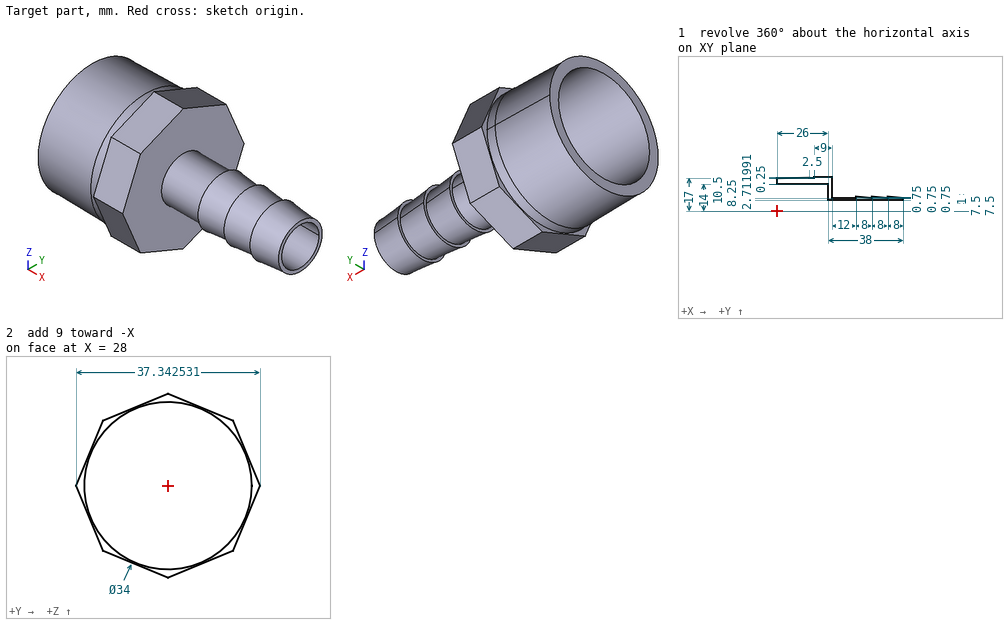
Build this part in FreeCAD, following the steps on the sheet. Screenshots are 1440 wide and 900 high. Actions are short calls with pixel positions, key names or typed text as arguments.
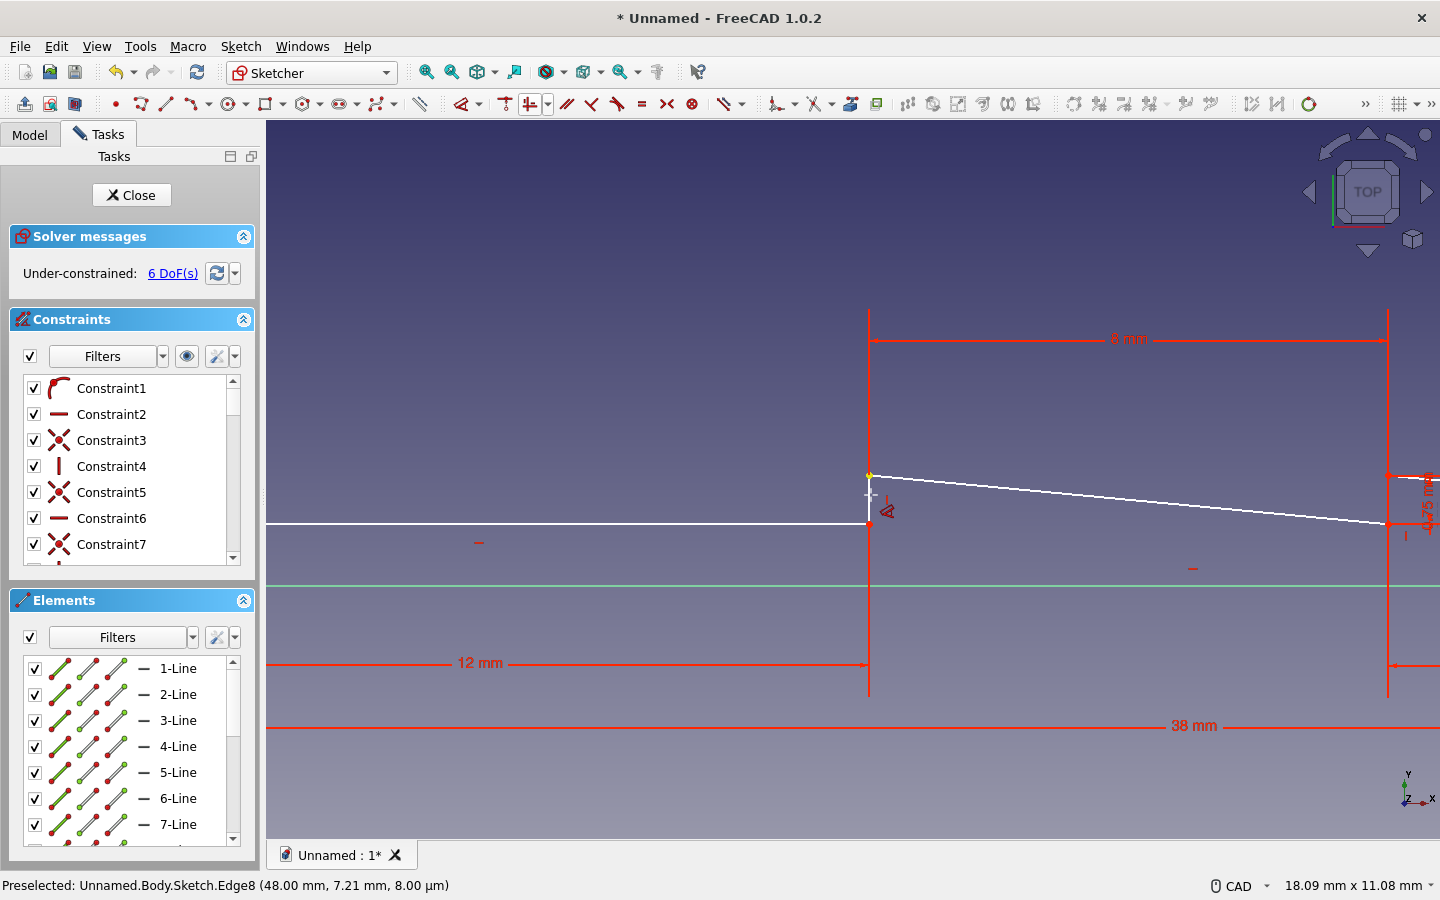
click(869, 490)
click(903, 500)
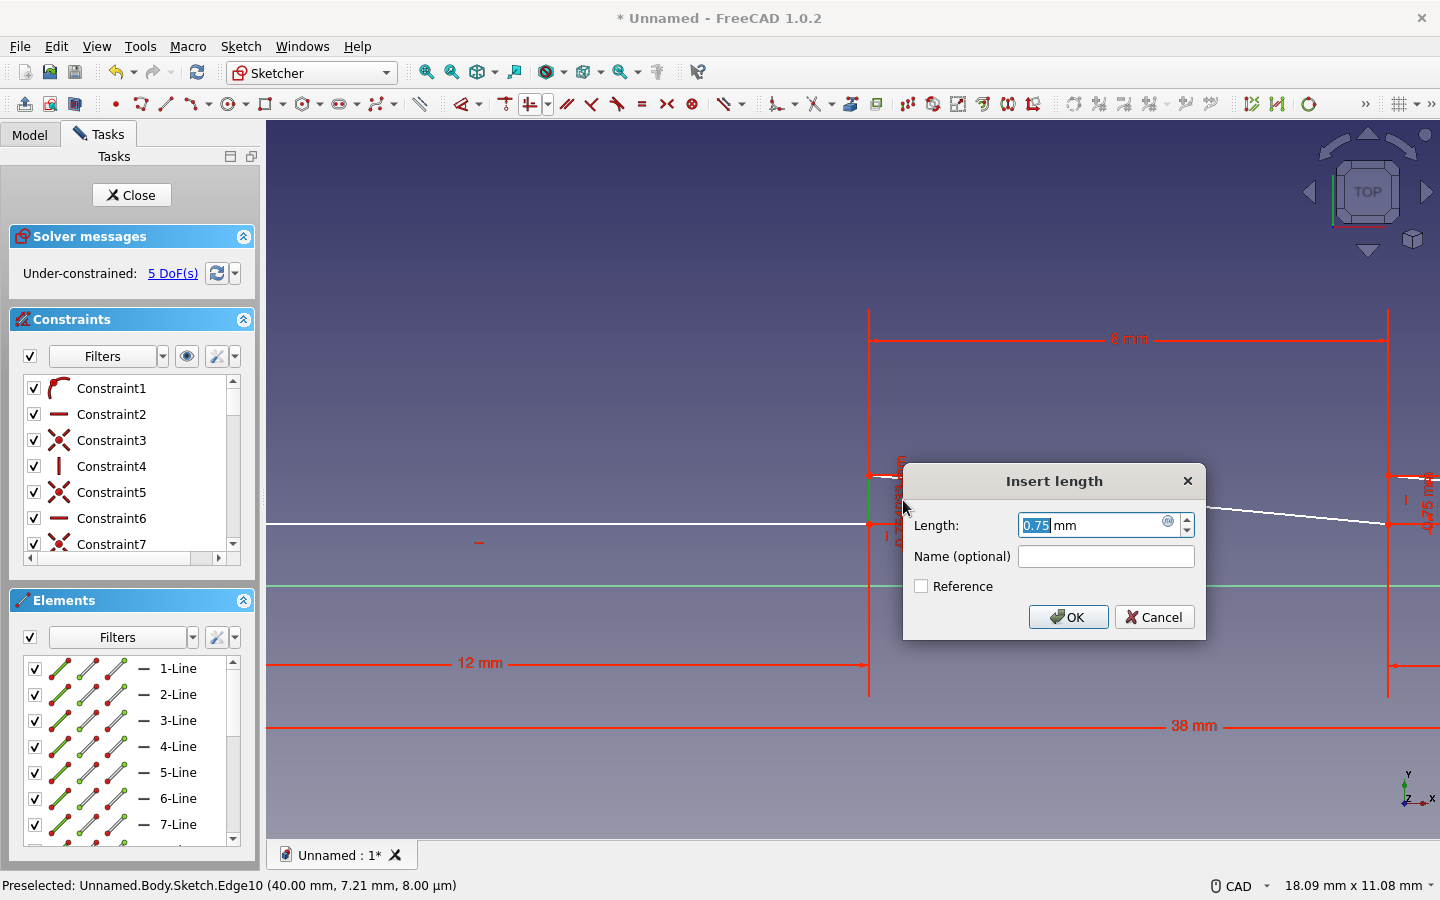
text(0.75)
key(Return)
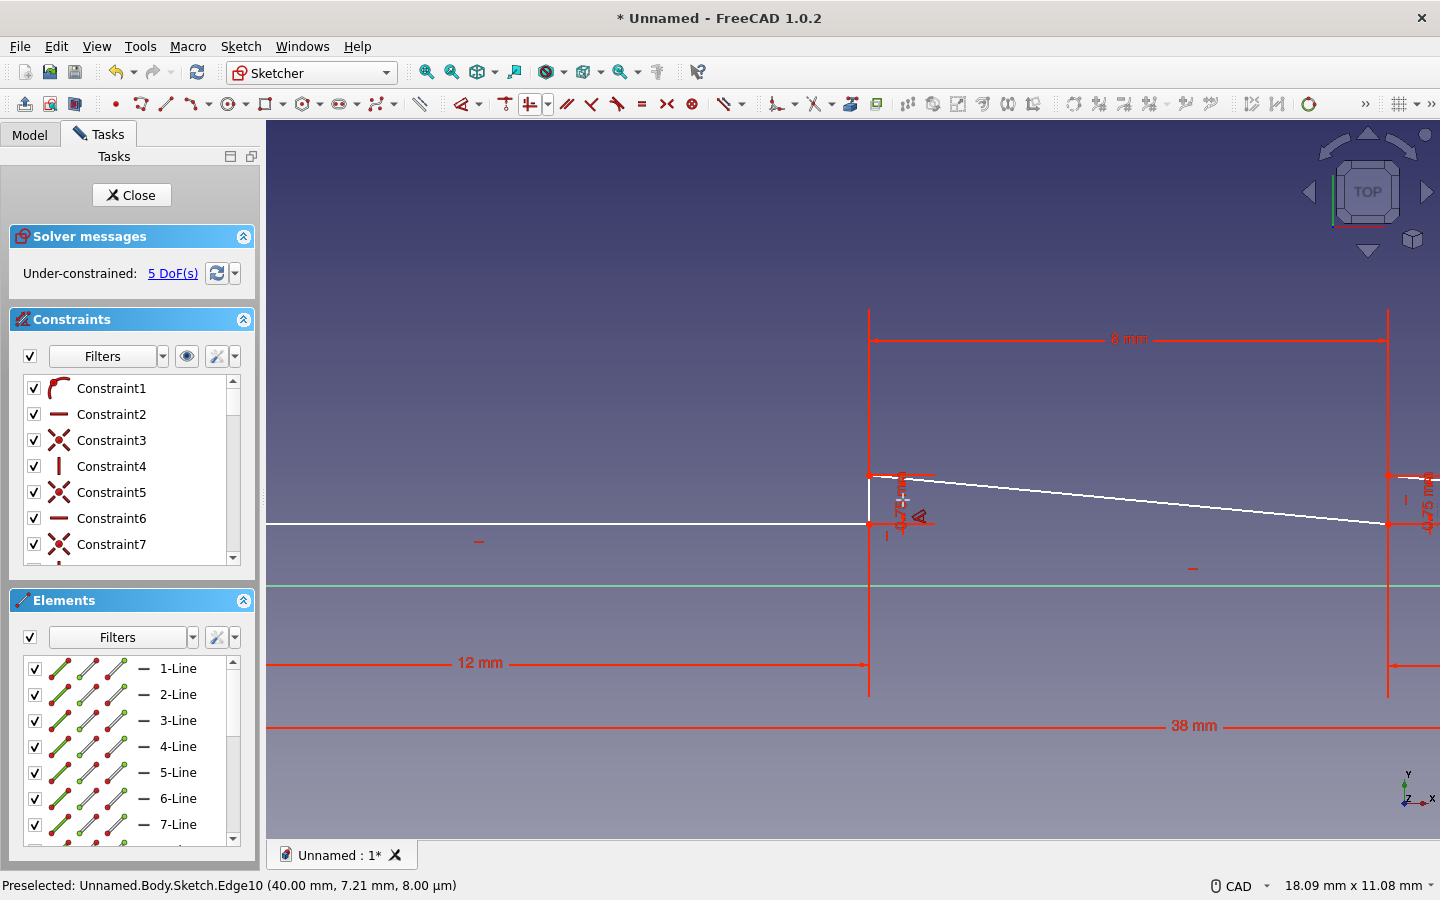
scroll(871, 495, down, 9)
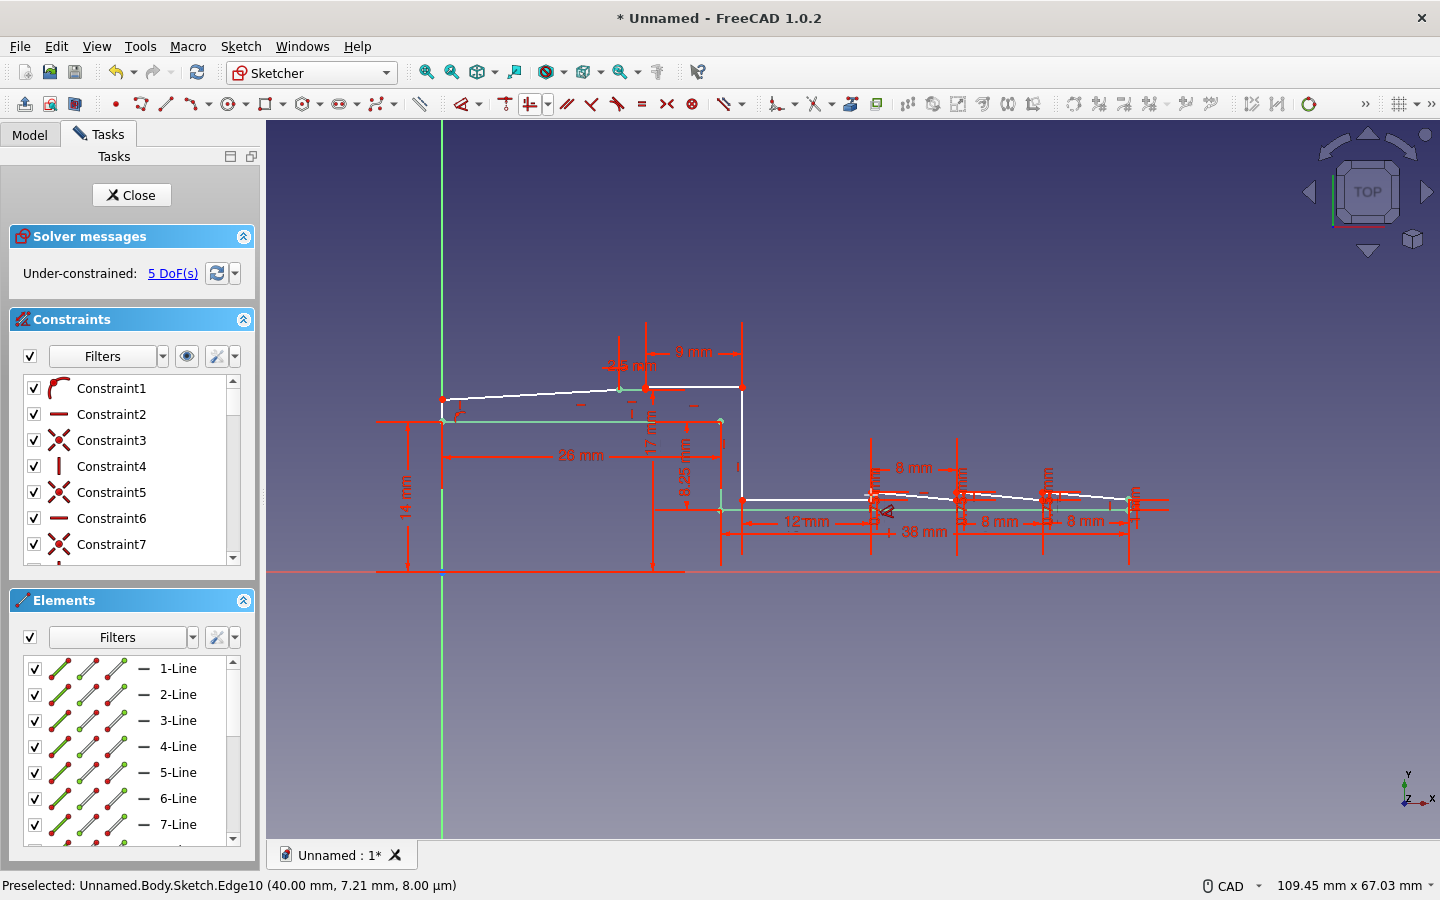
click(742, 466)
click(708, 404)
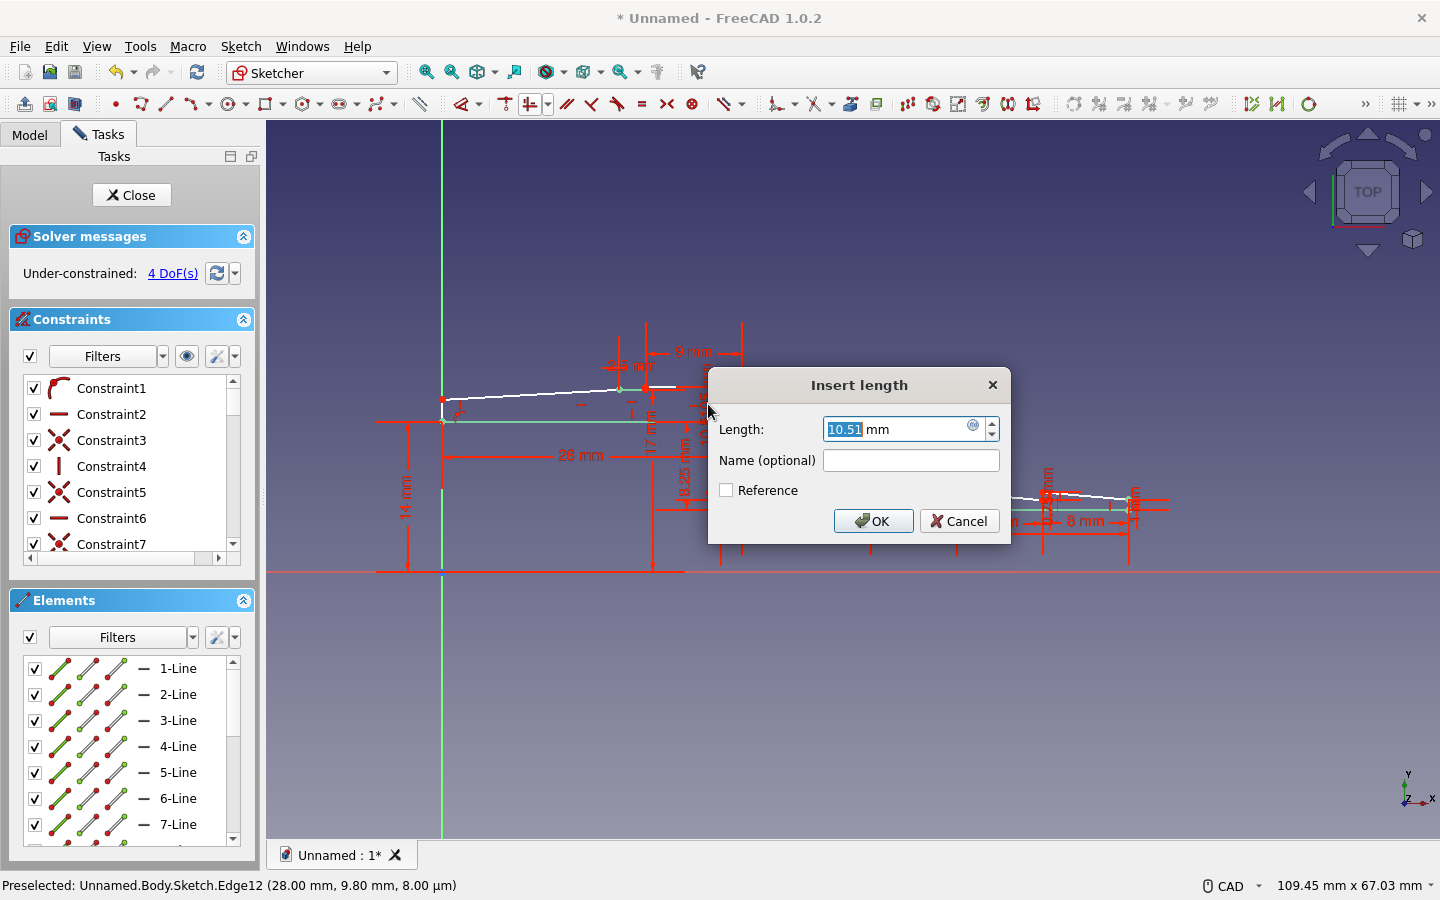
text(10.5)
key(Return)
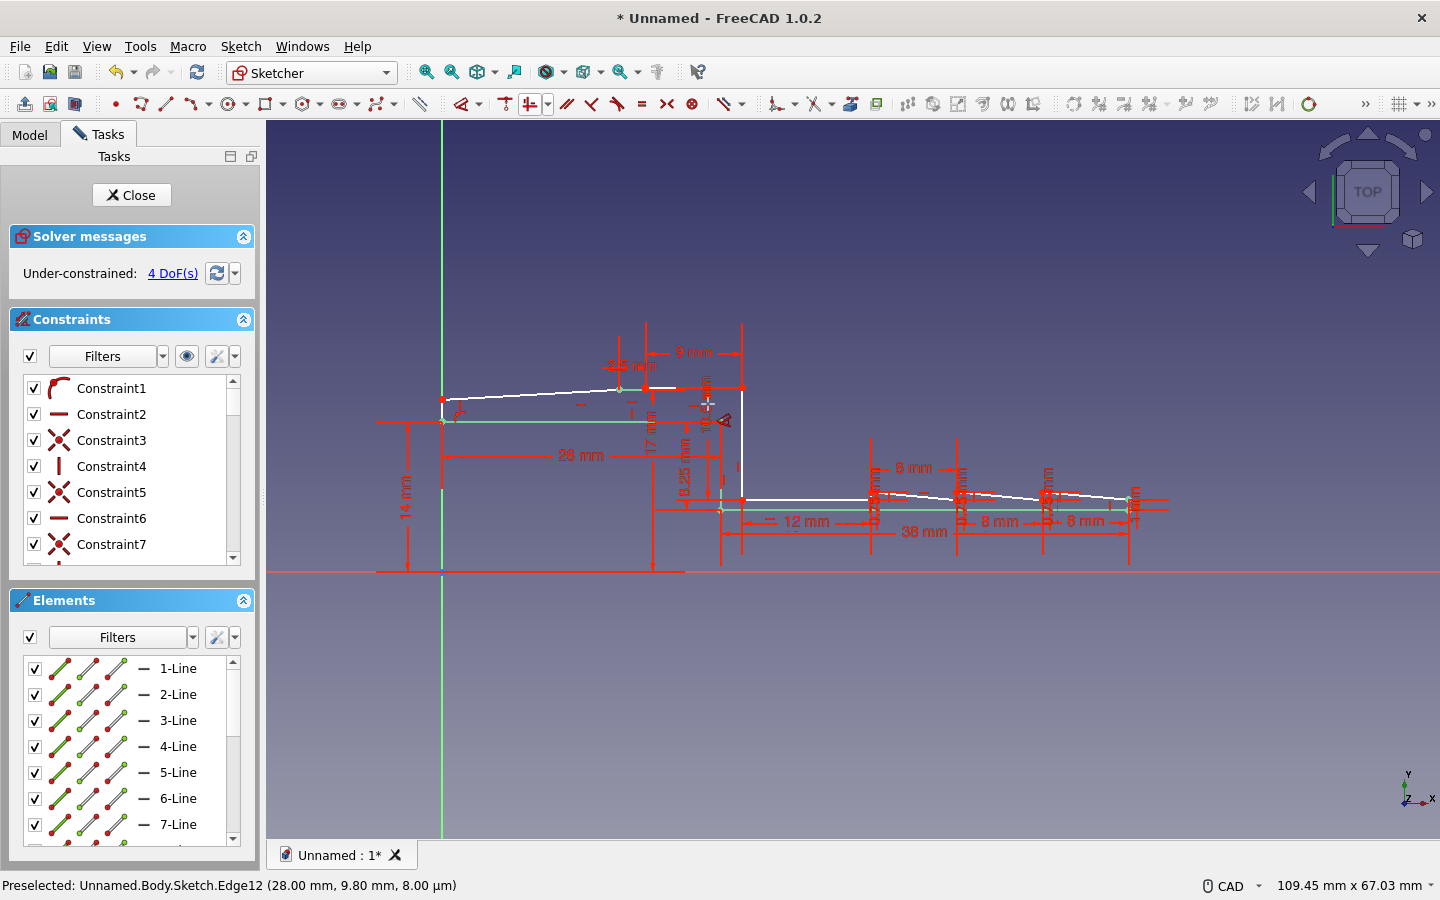
scroll(646, 389, up, 14)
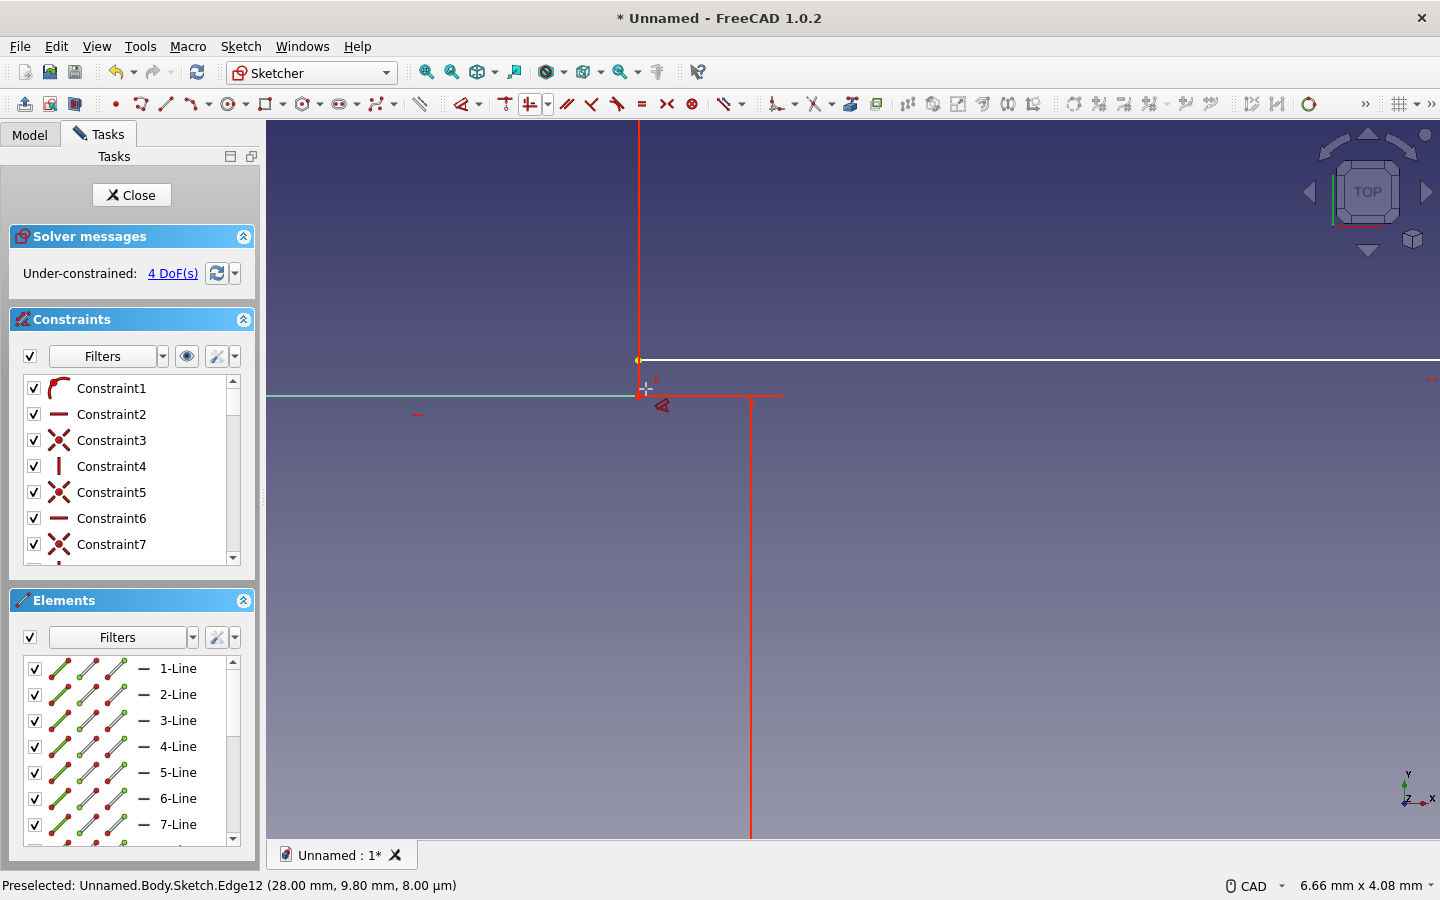
click(639, 378)
click(605, 378)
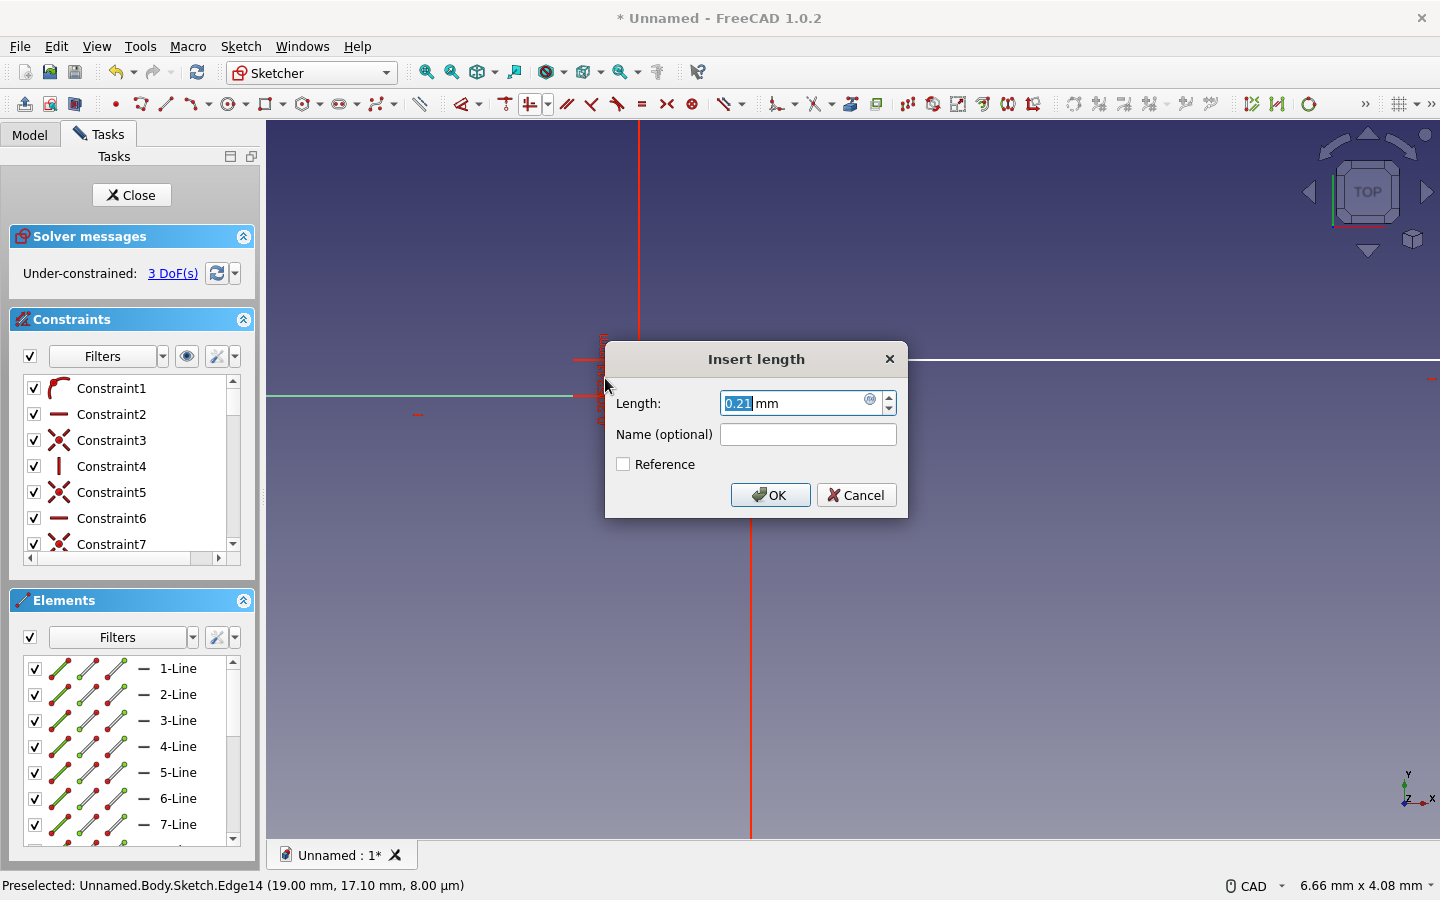
text(0.25)
key(Return)